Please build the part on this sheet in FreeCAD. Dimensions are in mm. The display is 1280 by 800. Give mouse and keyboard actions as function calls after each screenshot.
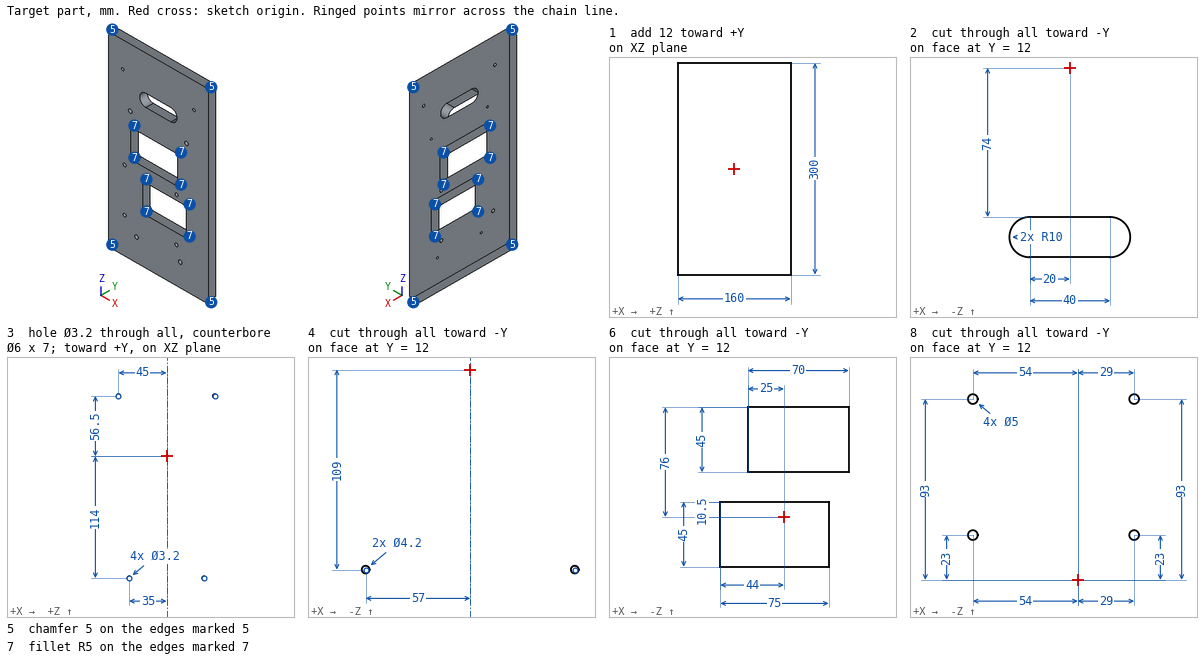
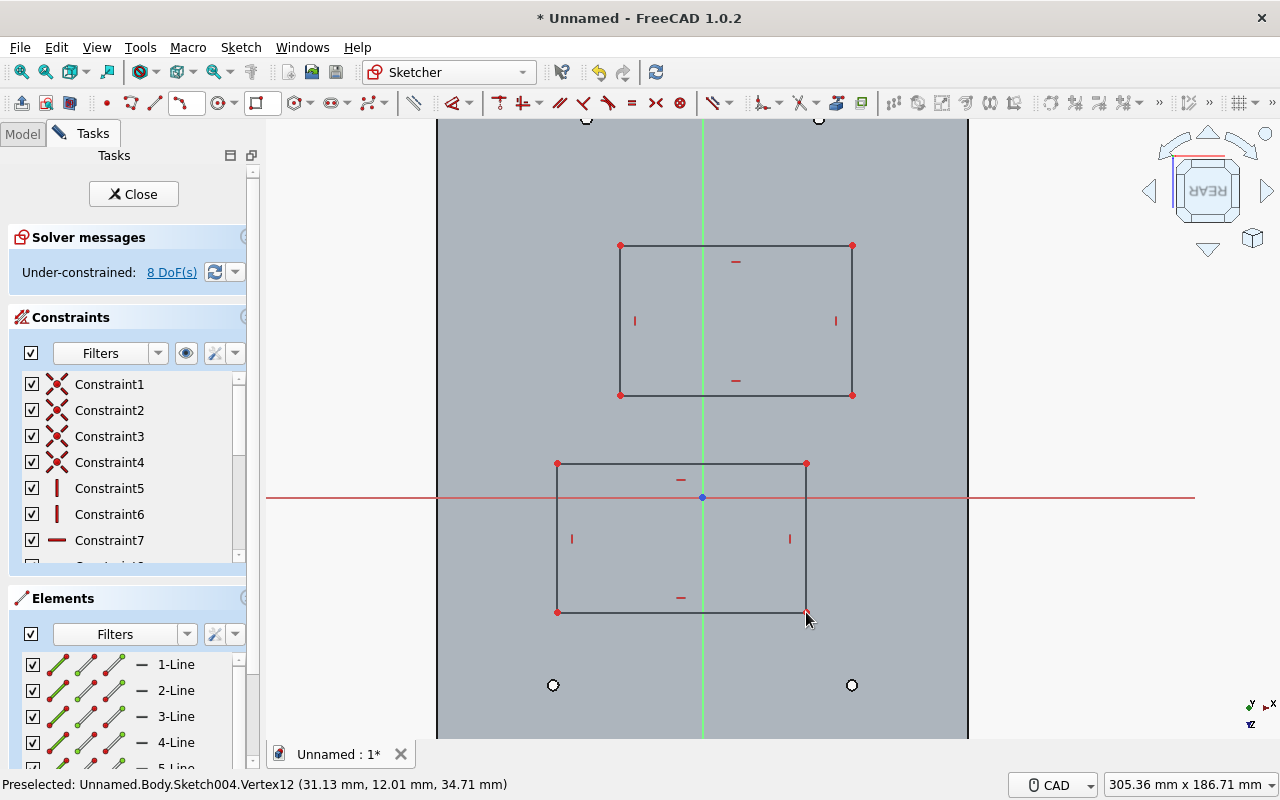
click(452, 104)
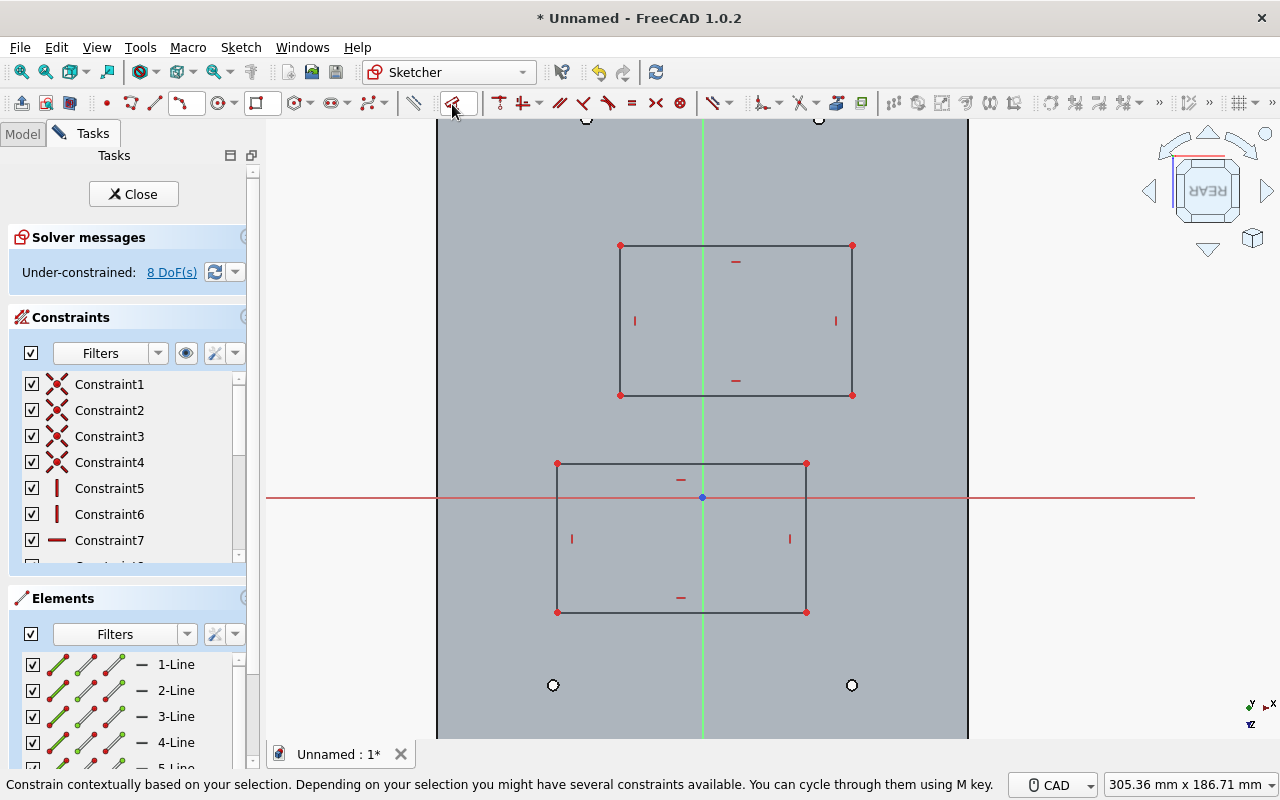
click(620, 291)
click(586, 321)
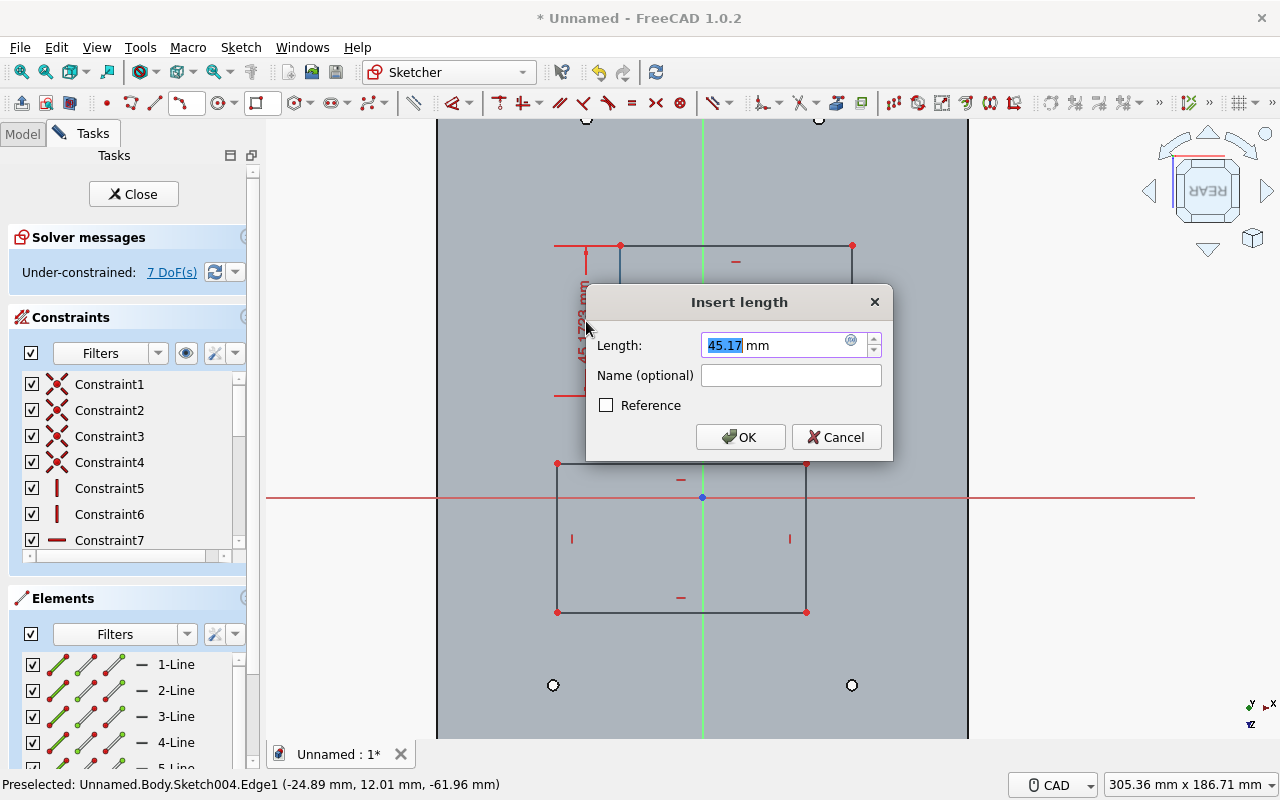
text(45)
key(Return)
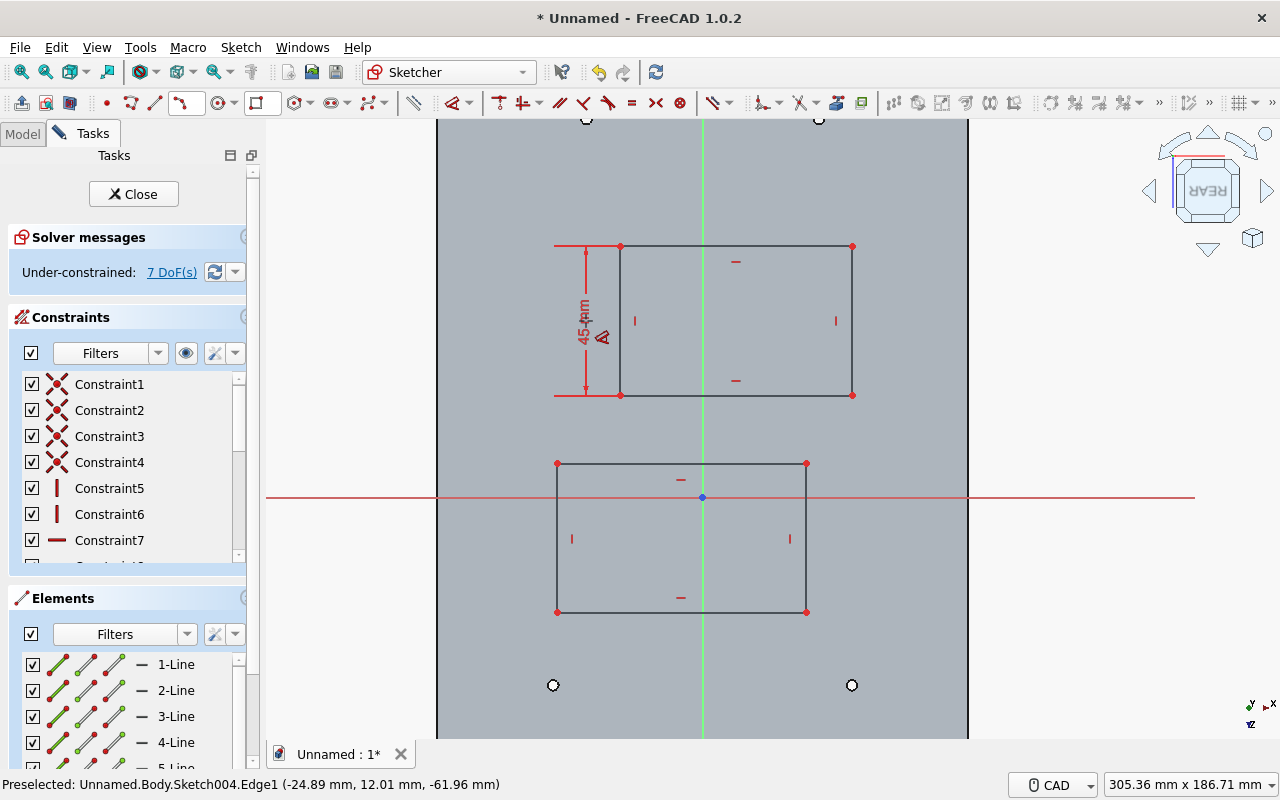
click(690, 396)
click(736, 362)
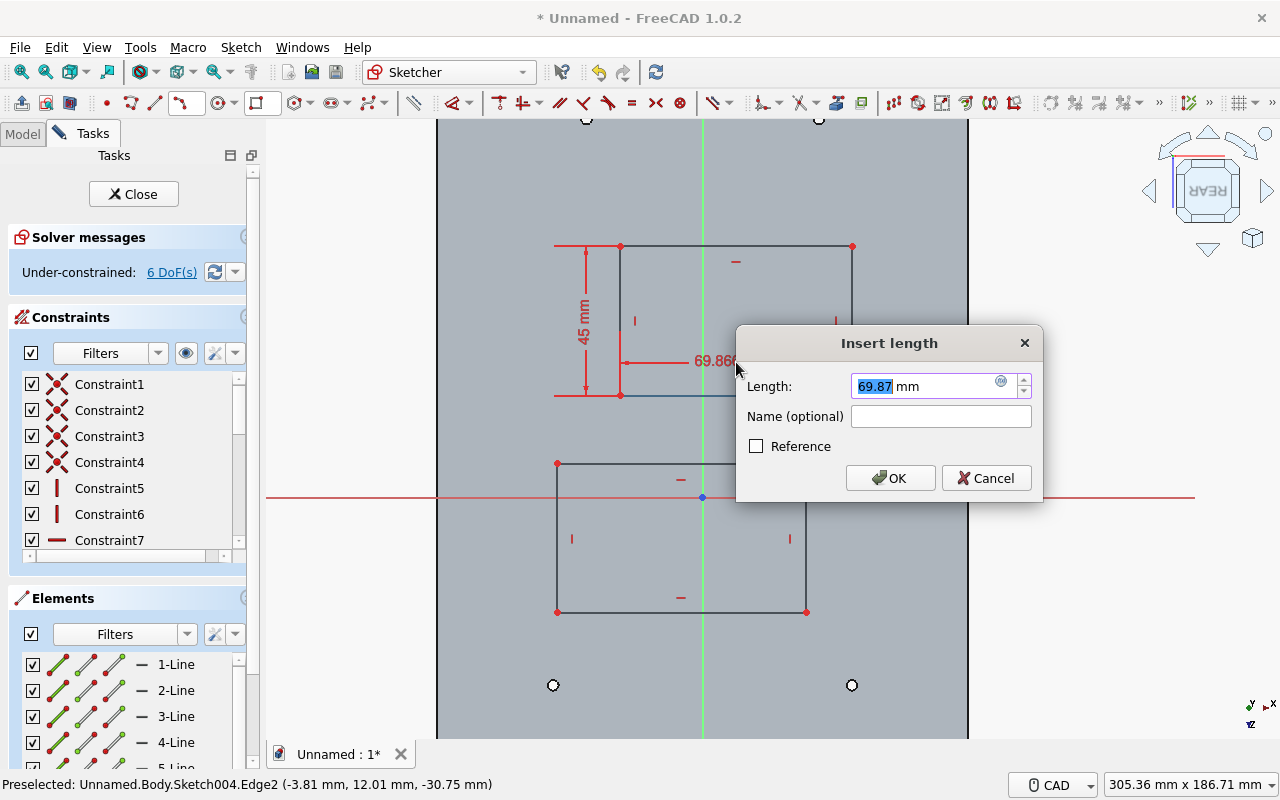
text(70)
key(Return)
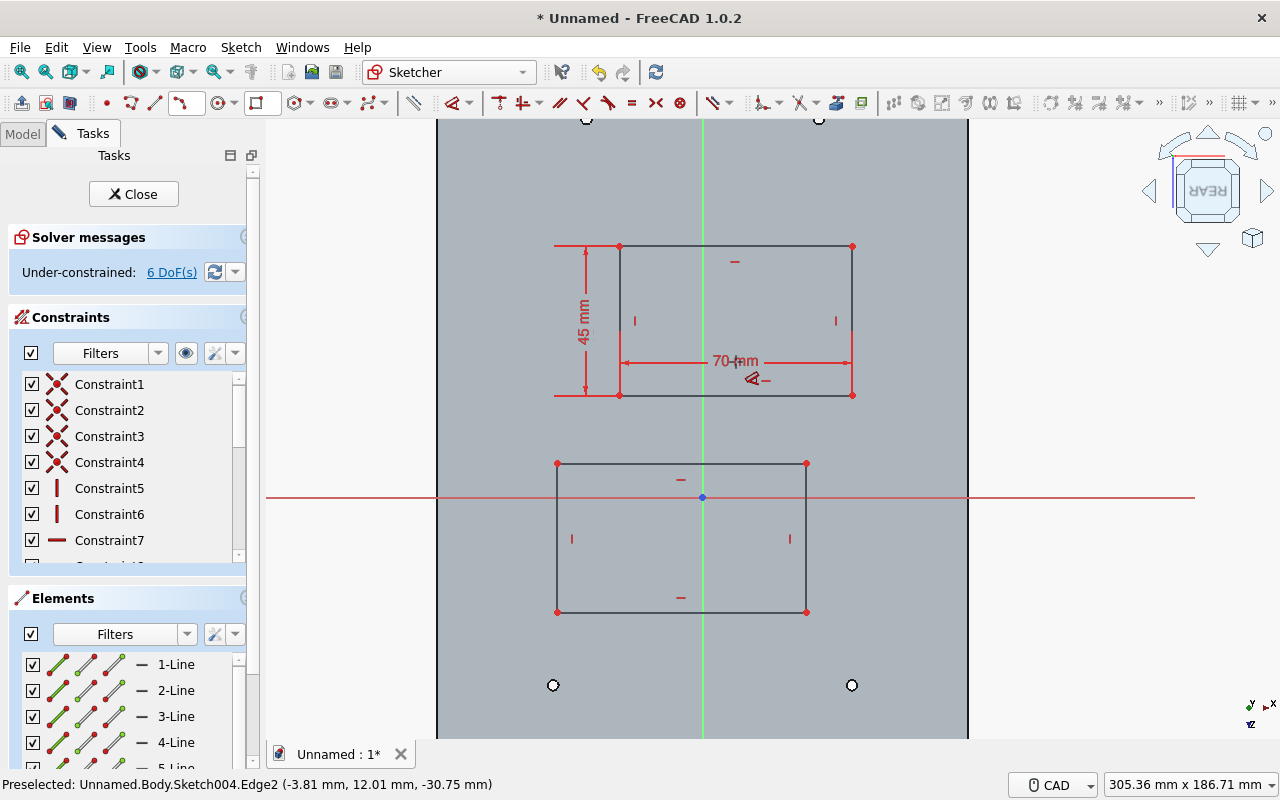
scroll(557, 509, up, 2)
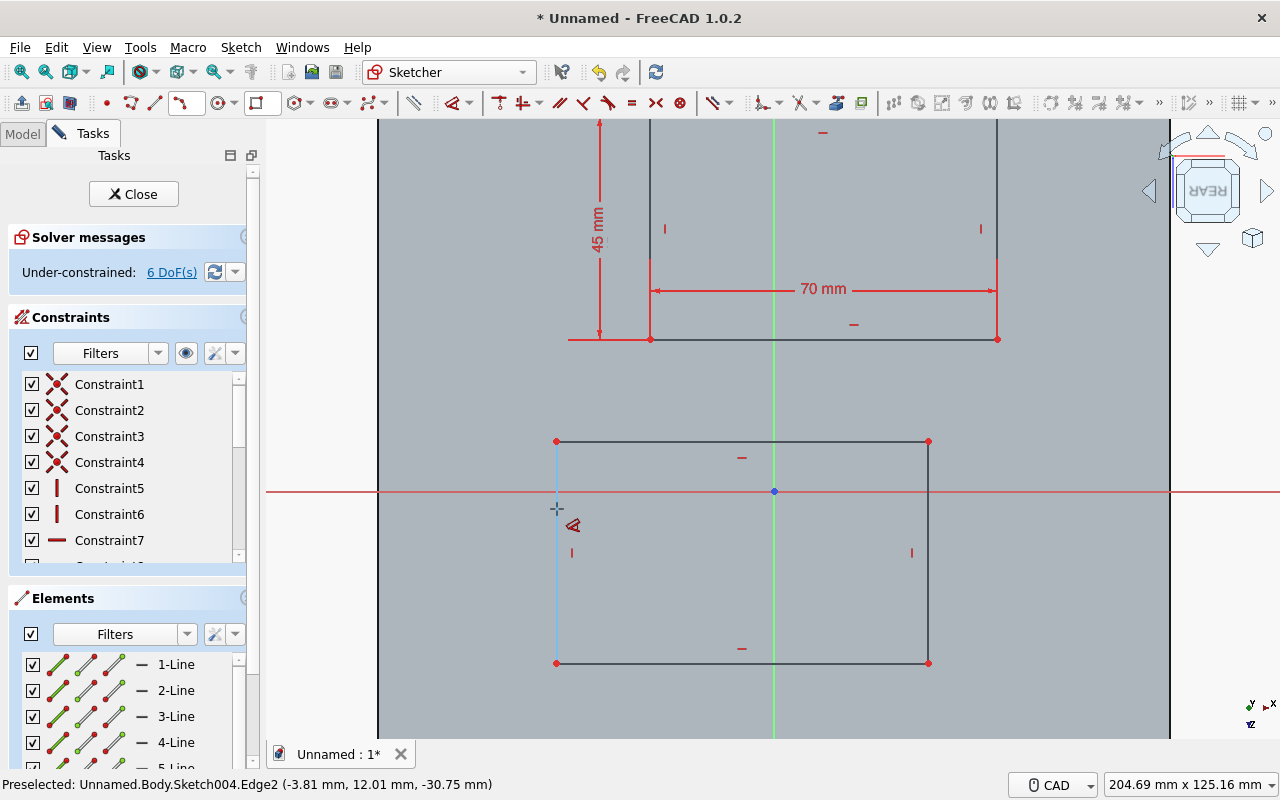
click(557, 508)
click(523, 553)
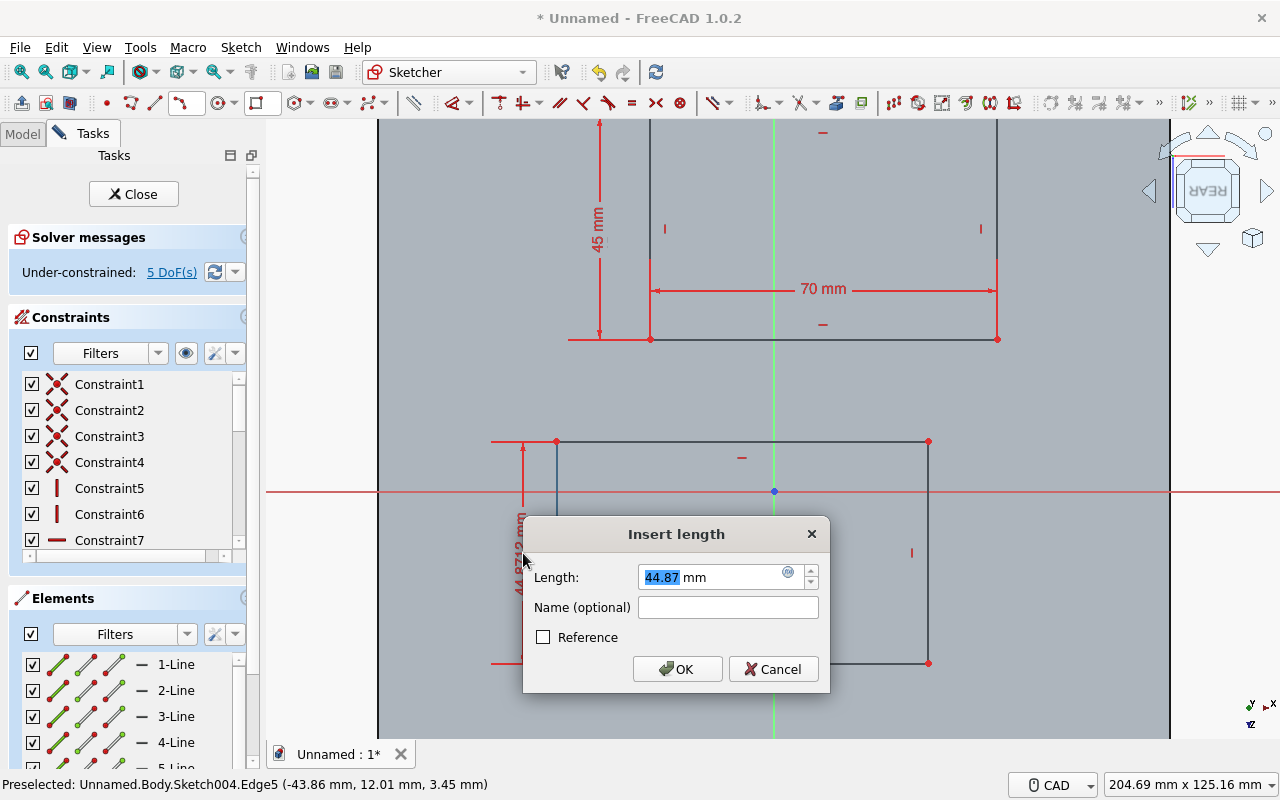
text(45)
key(Return)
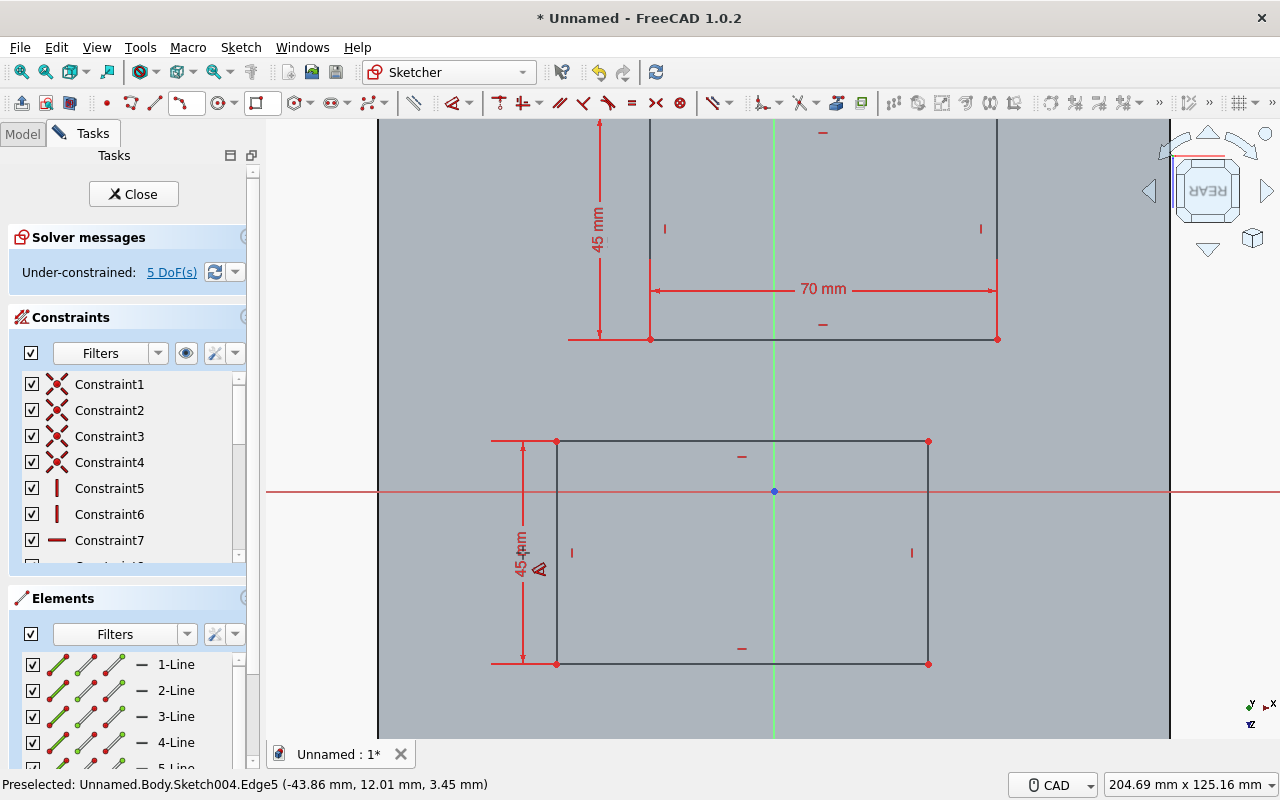
click(668, 664)
click(743, 698)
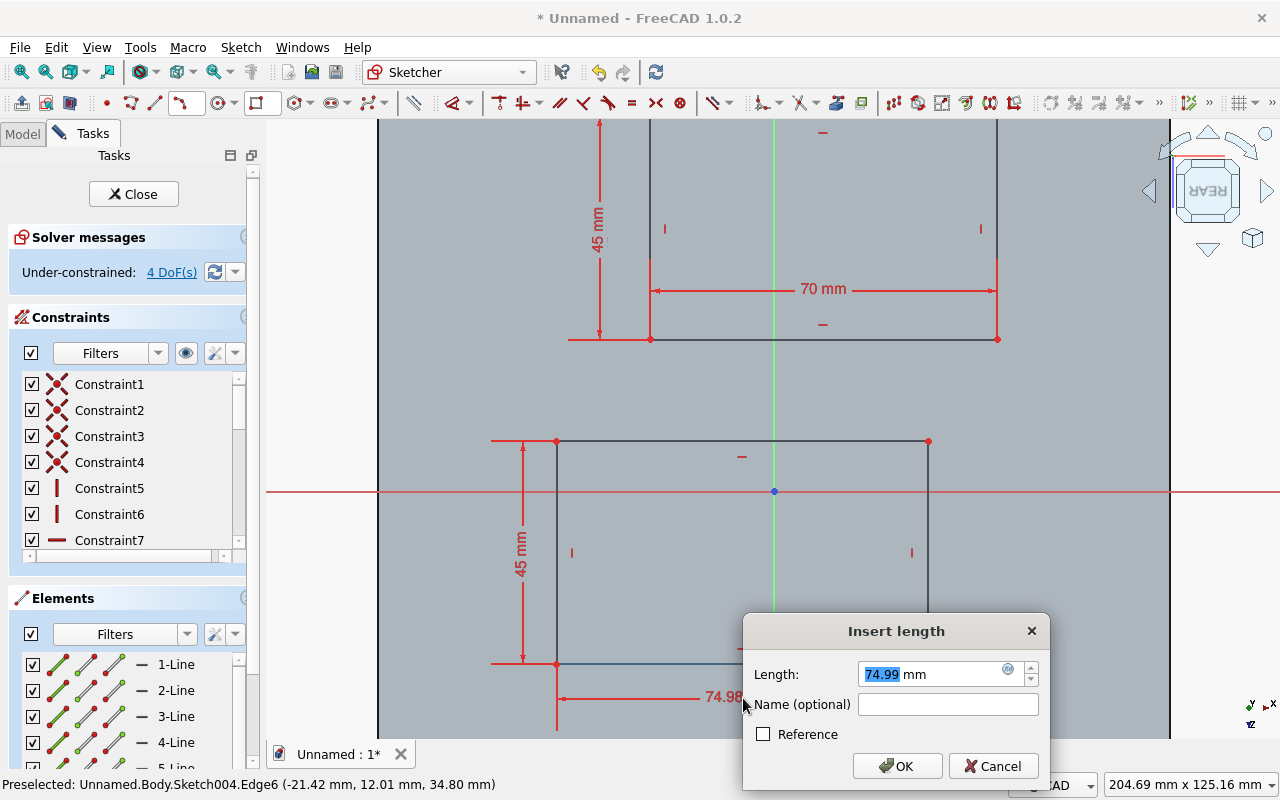
text(75)
key(Return)